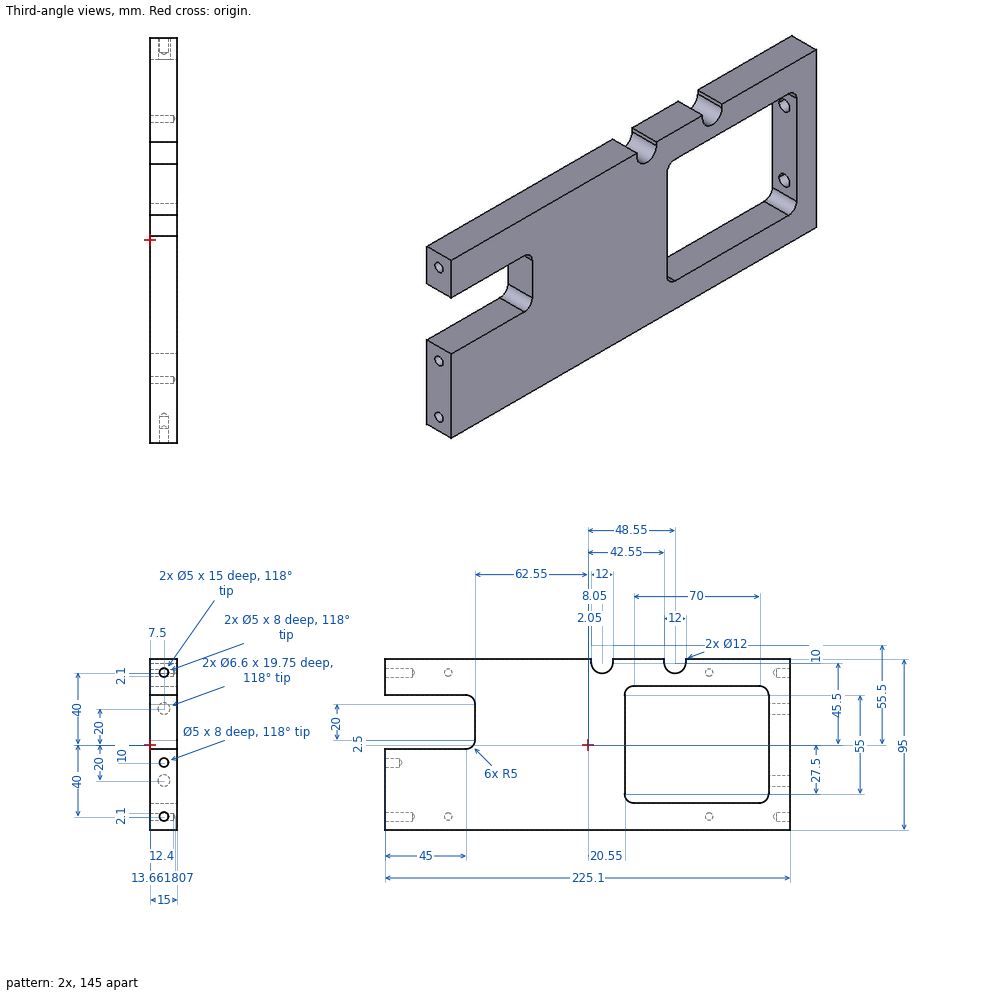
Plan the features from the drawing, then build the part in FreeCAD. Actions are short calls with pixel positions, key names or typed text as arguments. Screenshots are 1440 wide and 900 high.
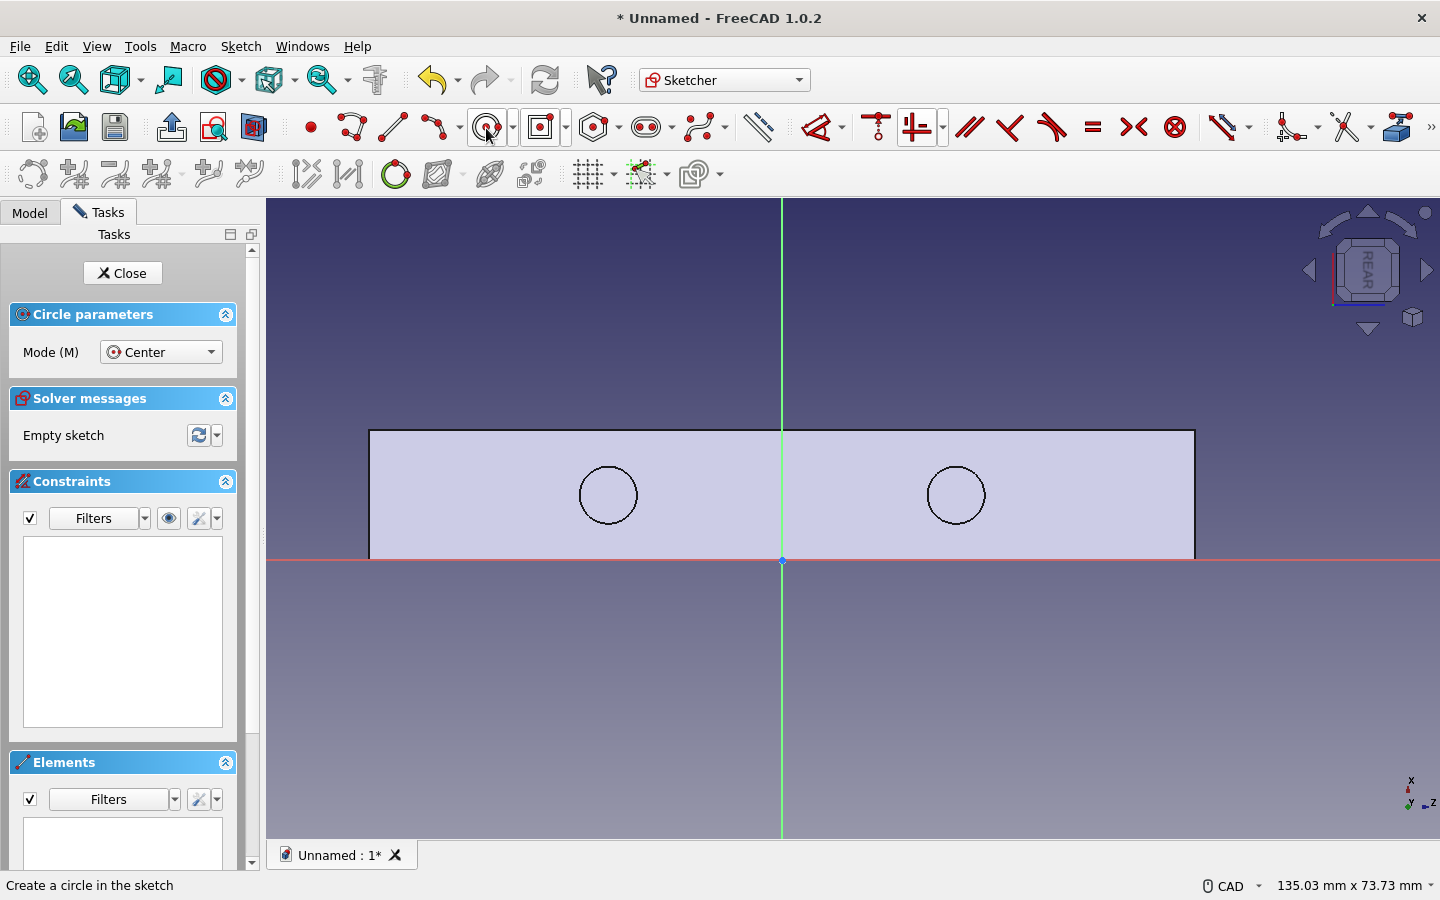
click(1130, 495)
move(1145, 480)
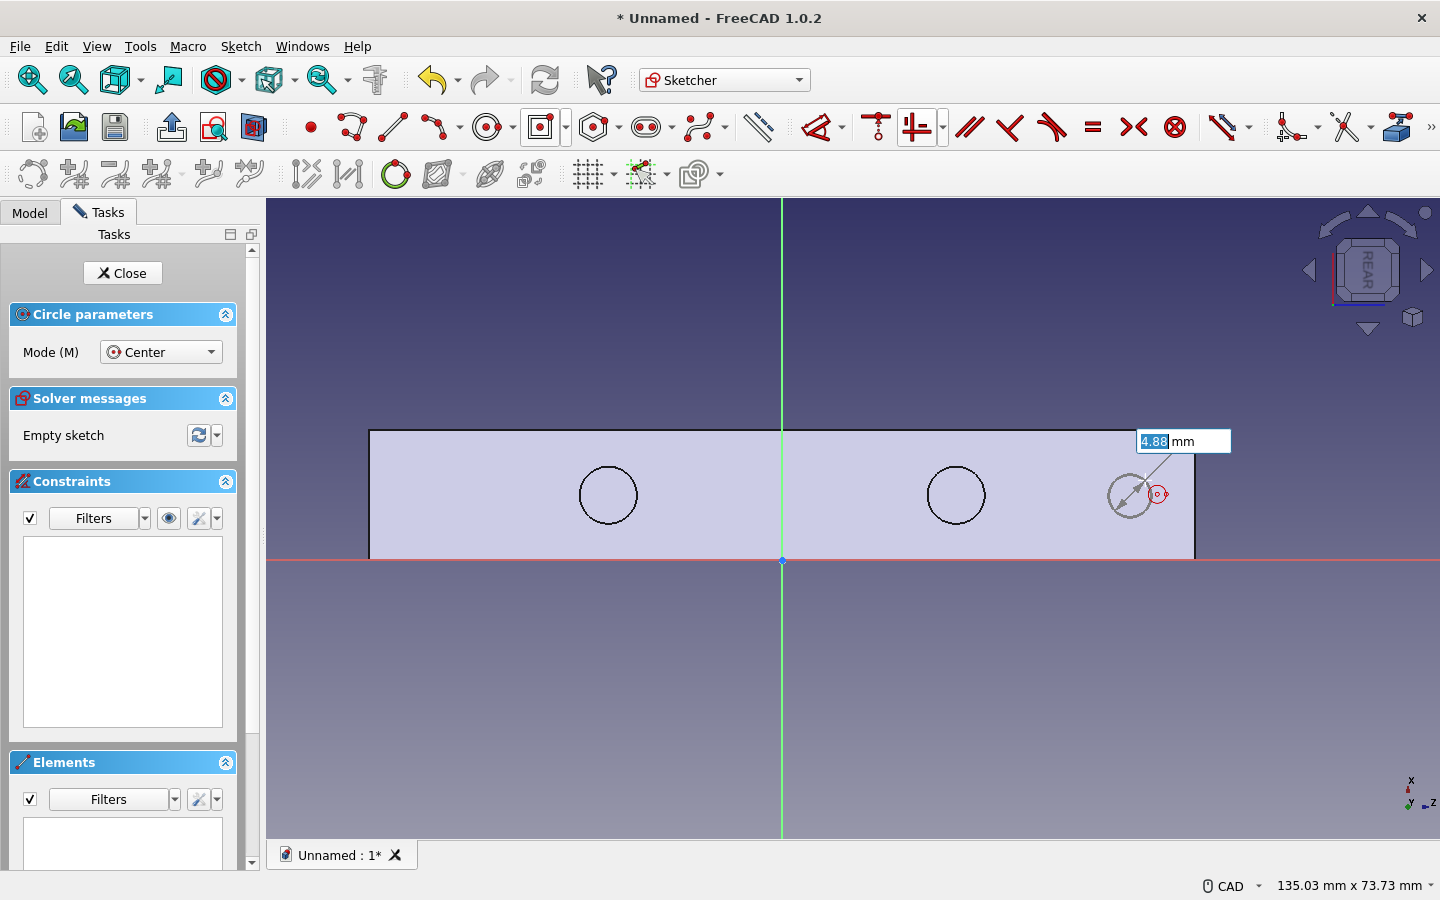
text(5)
key(Return)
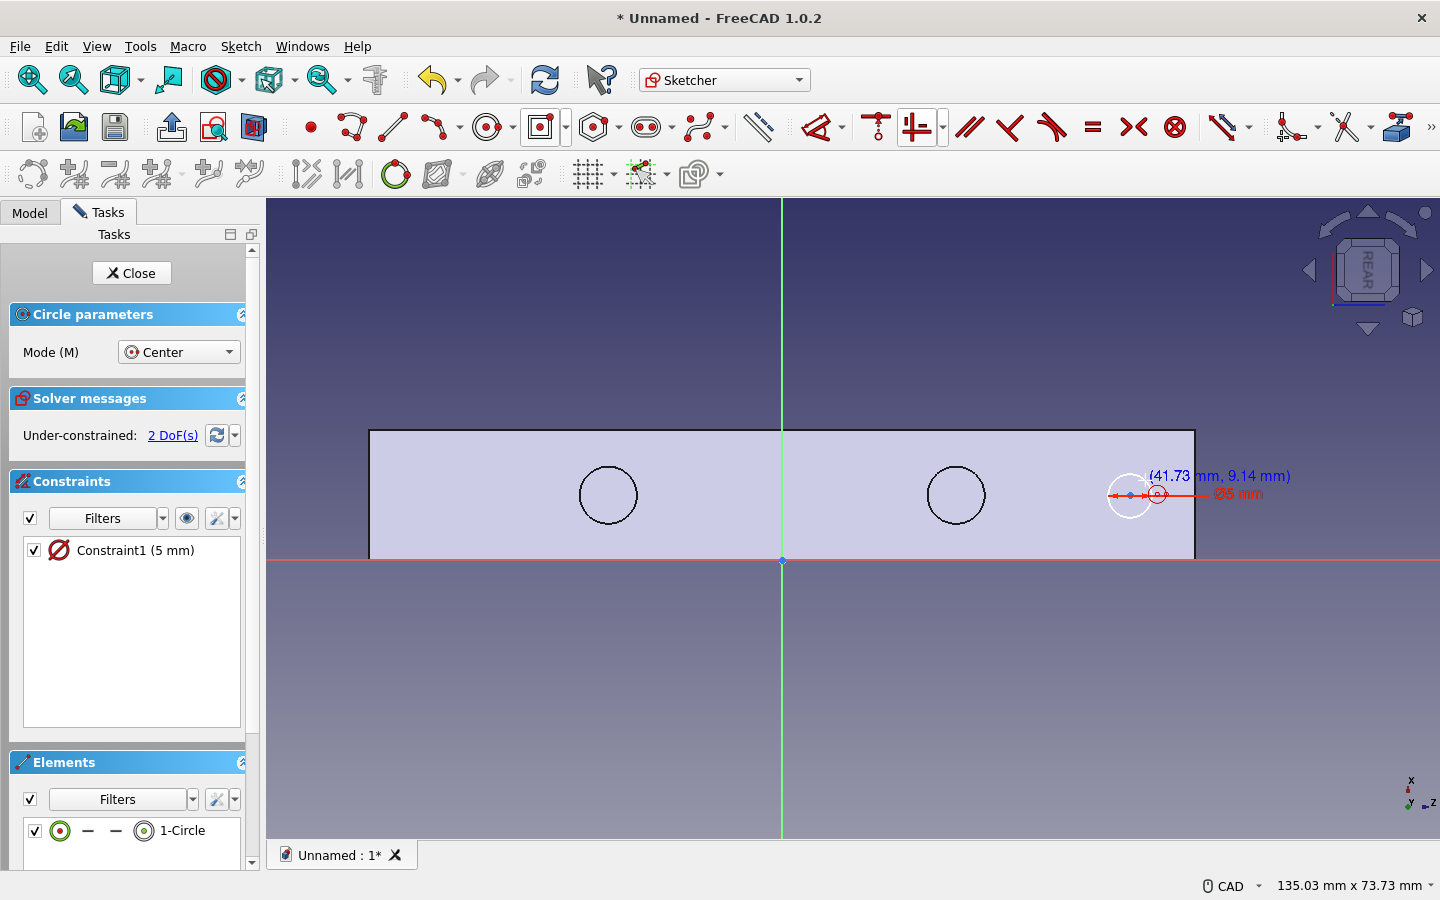
click(434, 495)
move(450, 480)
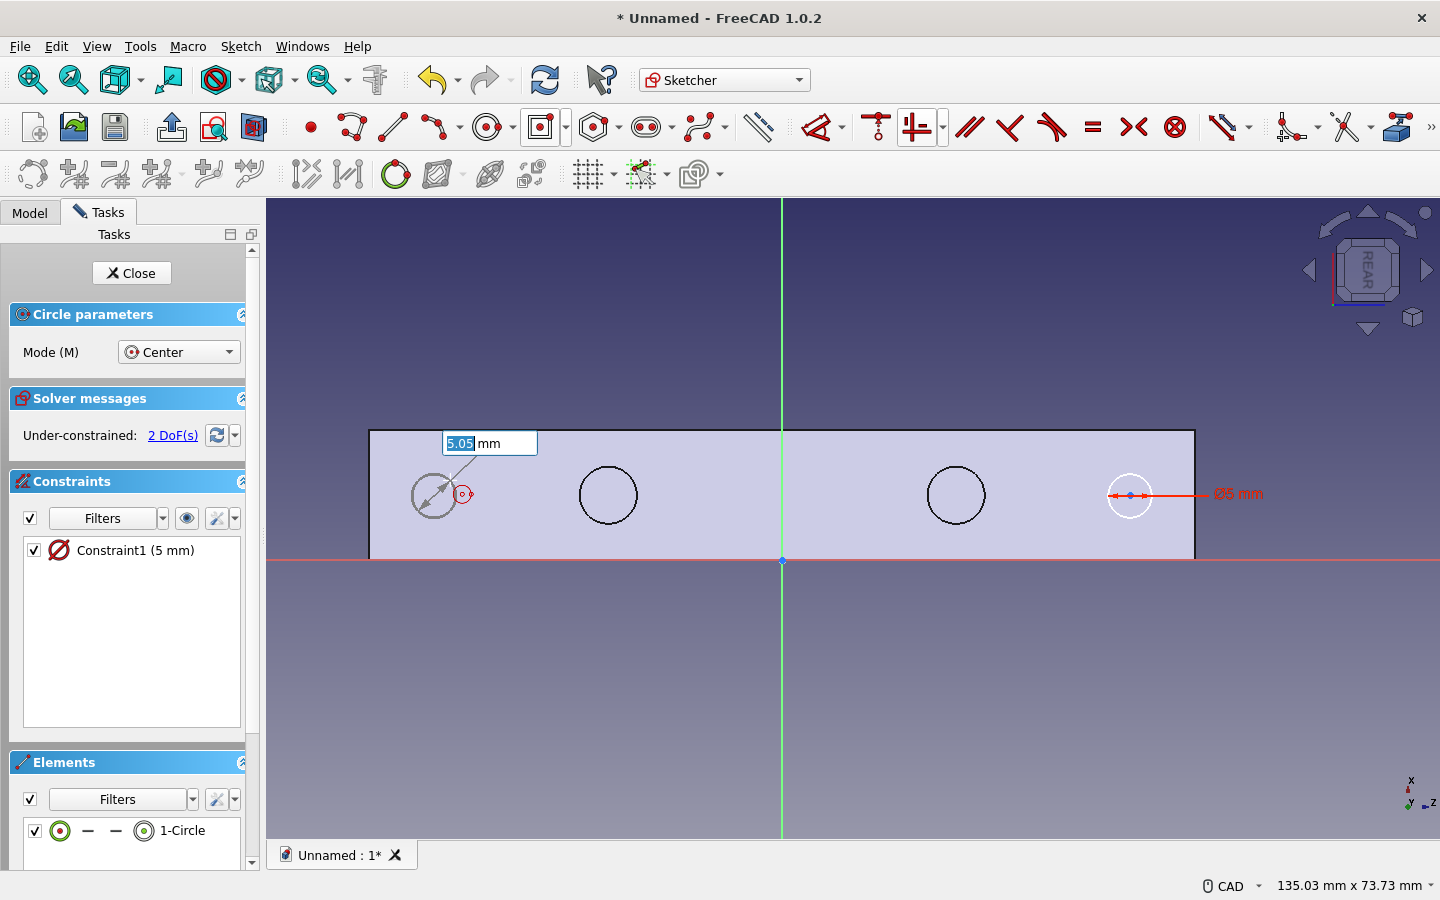
text(5)
key(Return)
key(Escape)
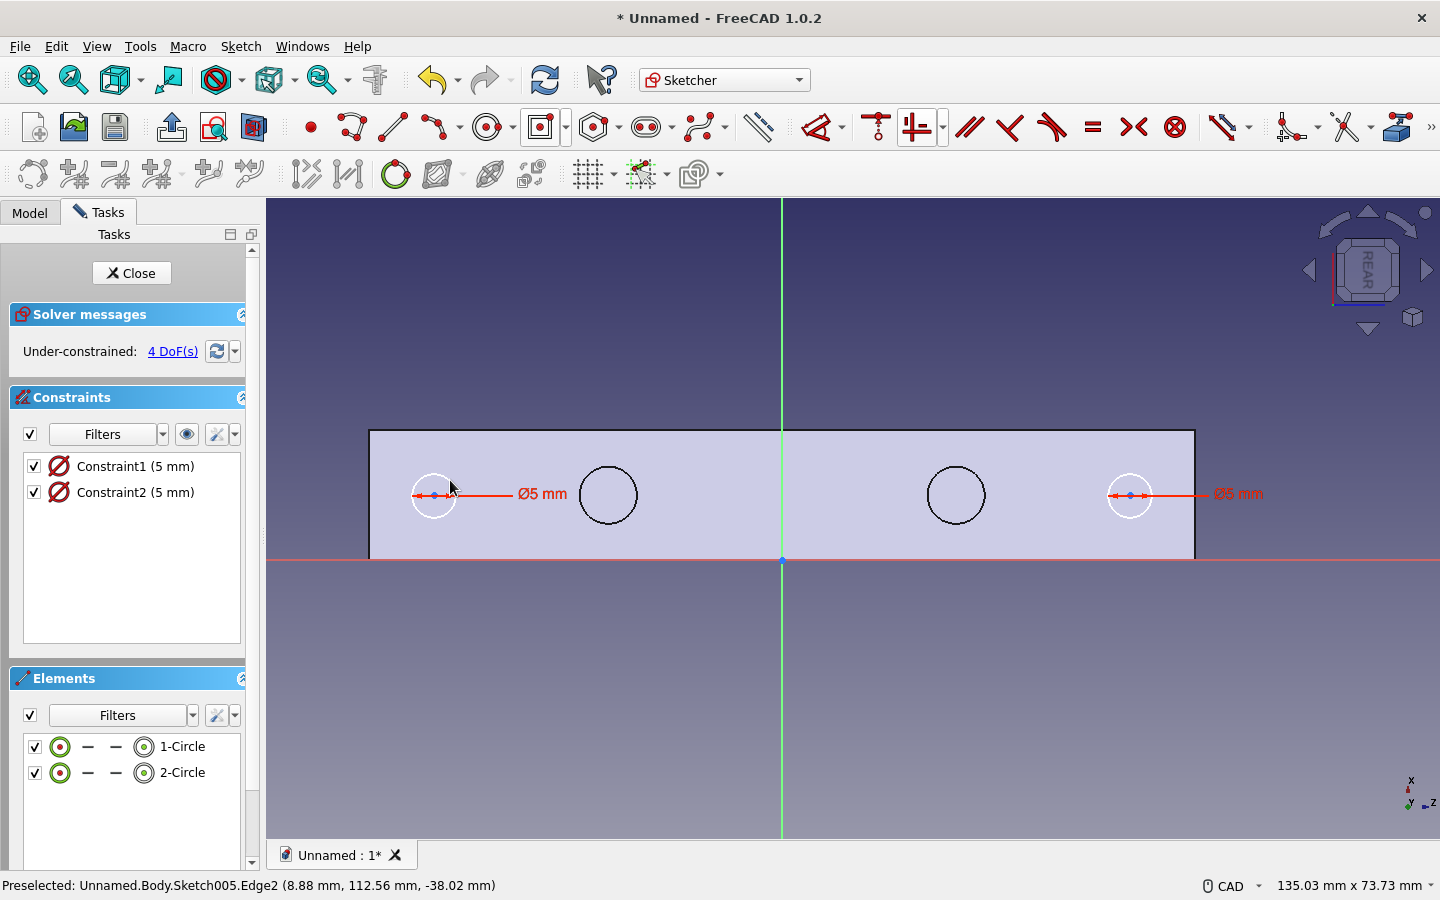
click(1130, 496)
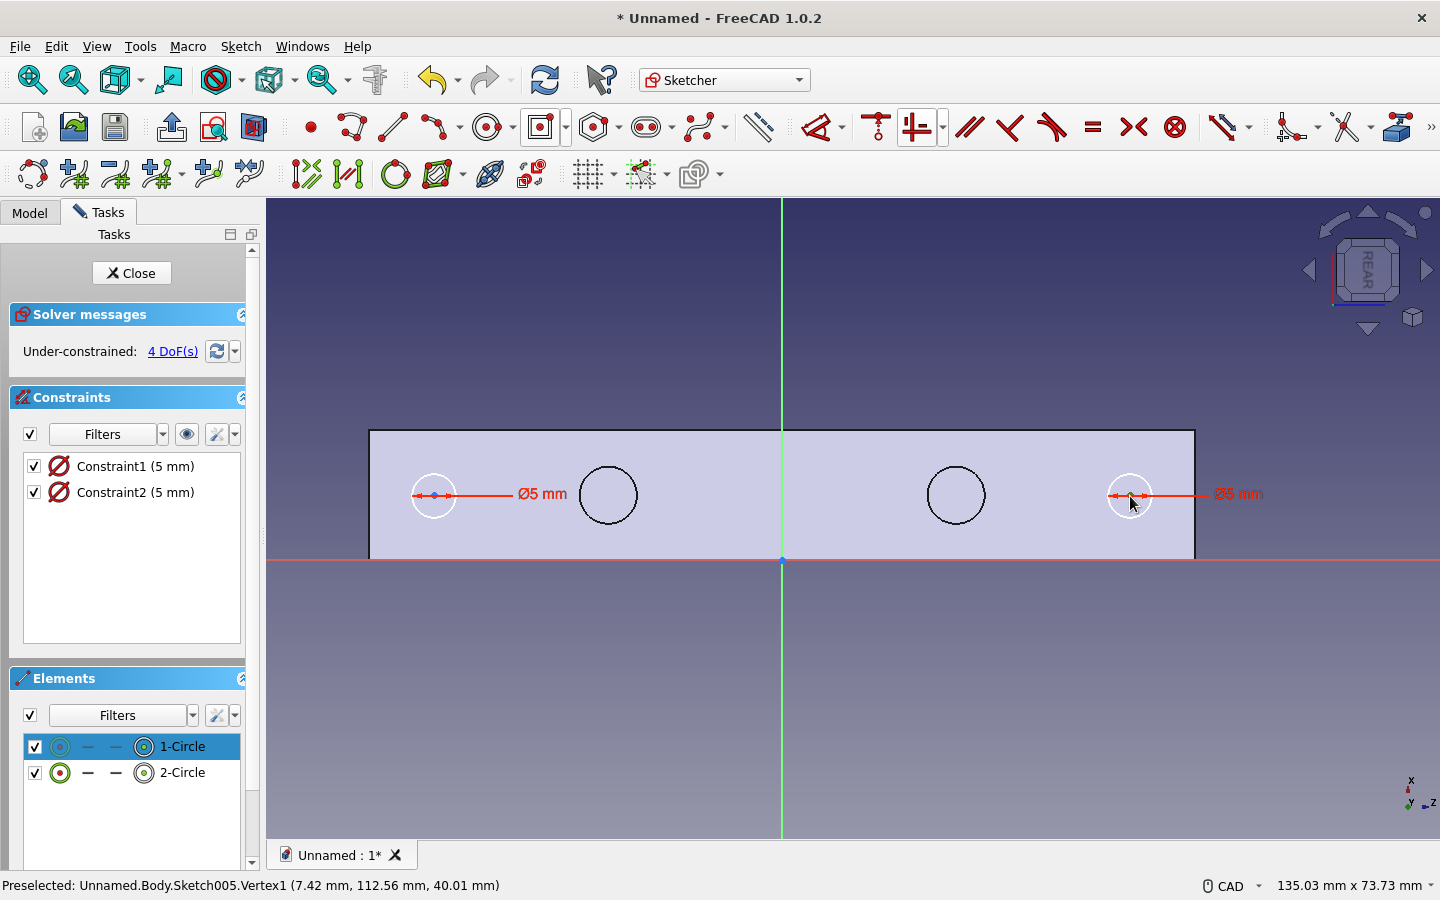
click(434, 496)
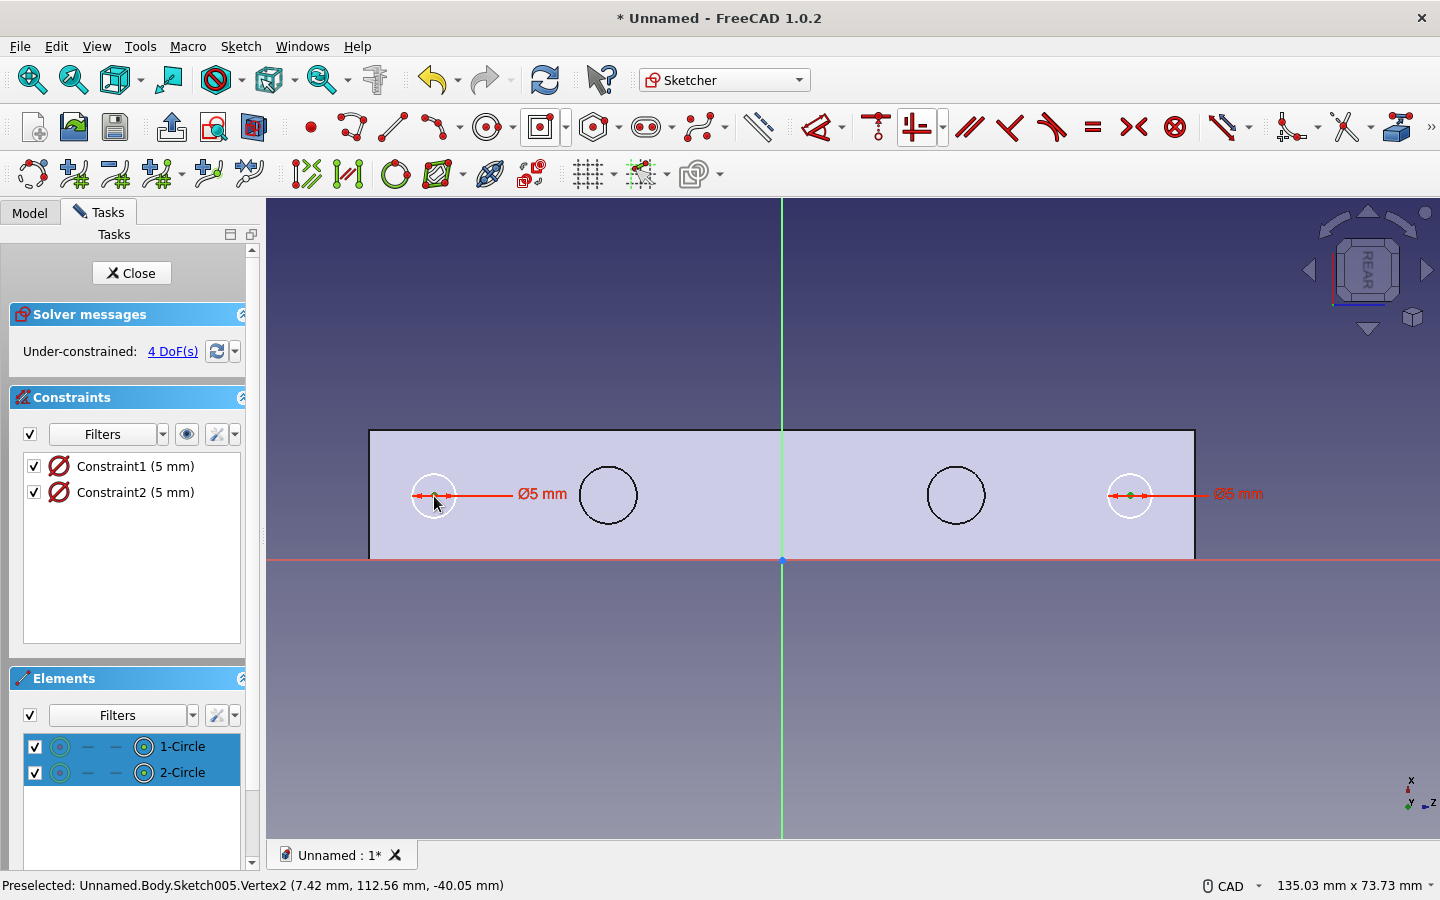
click(942, 128)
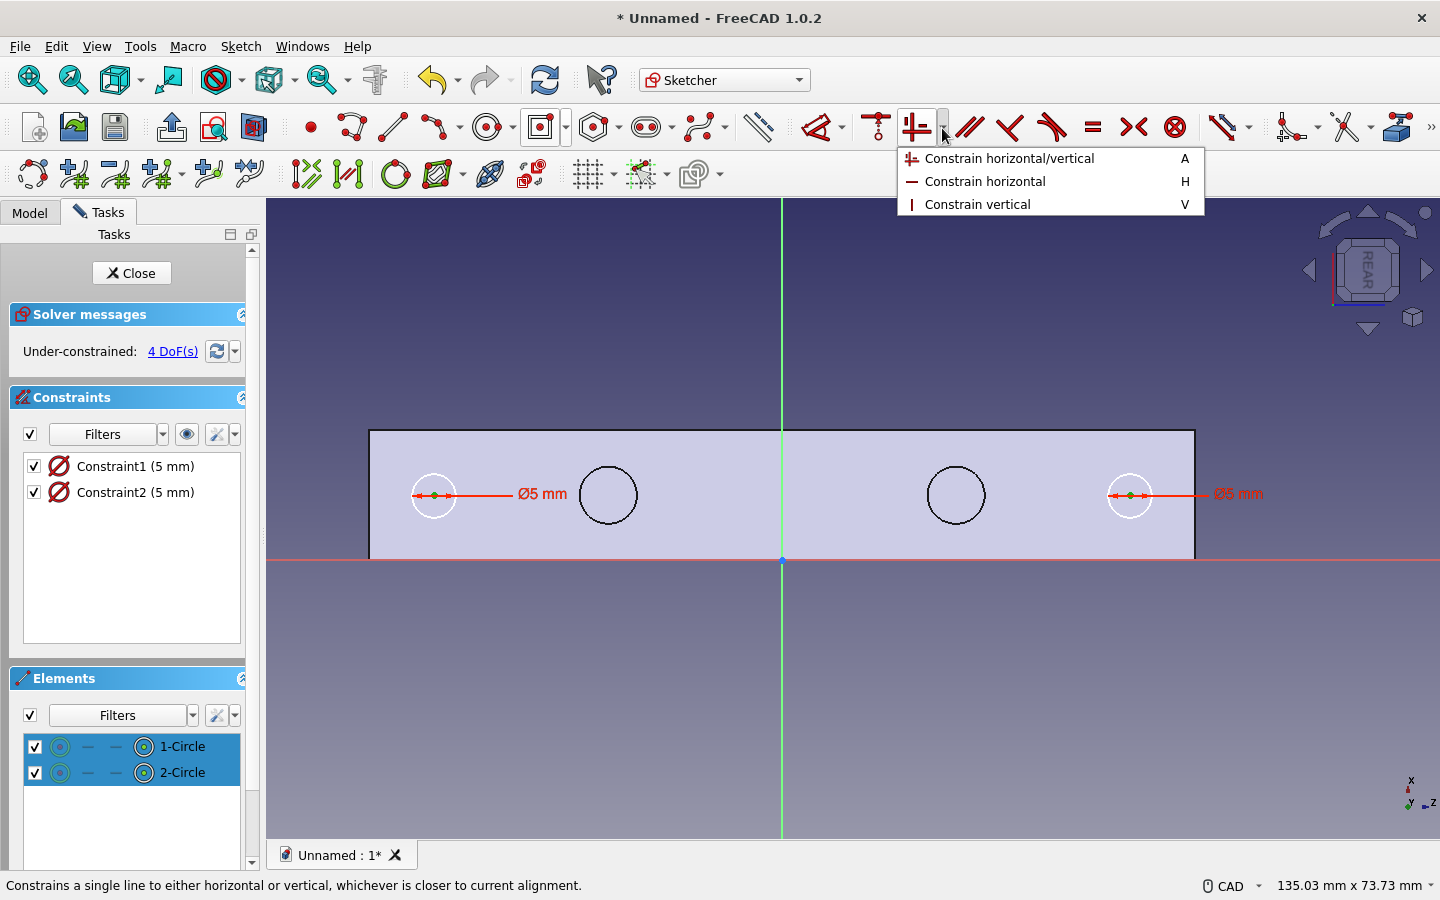
click(1051, 182)